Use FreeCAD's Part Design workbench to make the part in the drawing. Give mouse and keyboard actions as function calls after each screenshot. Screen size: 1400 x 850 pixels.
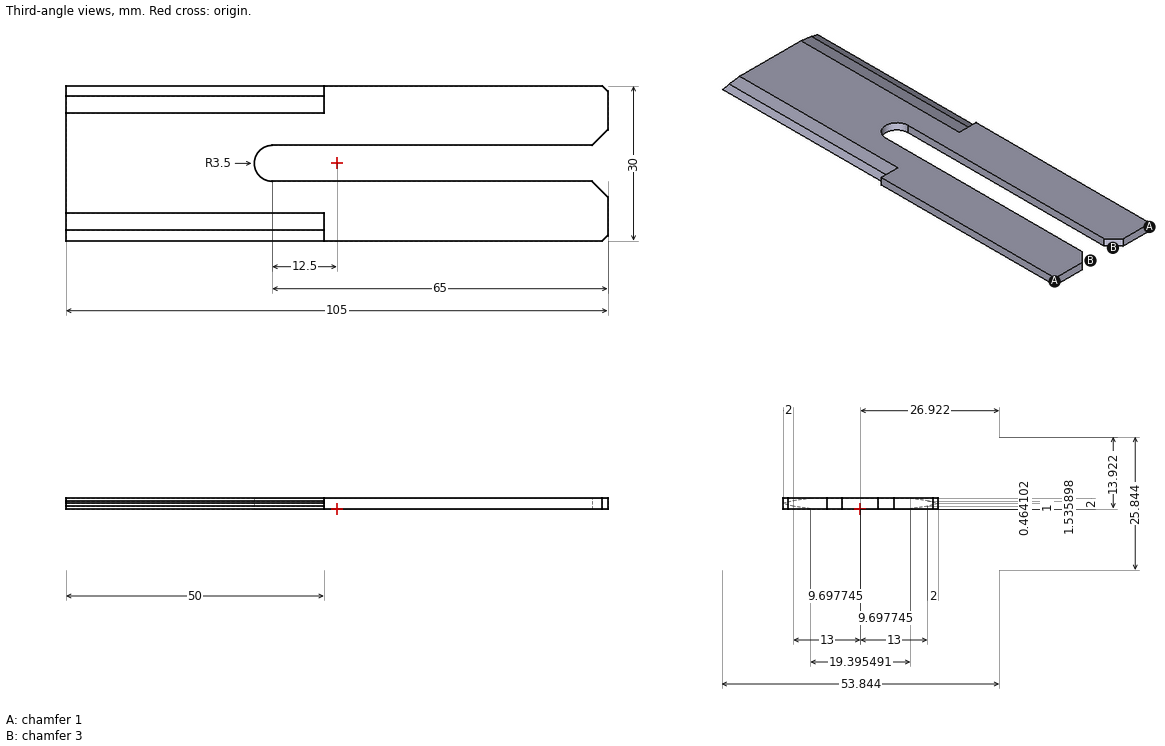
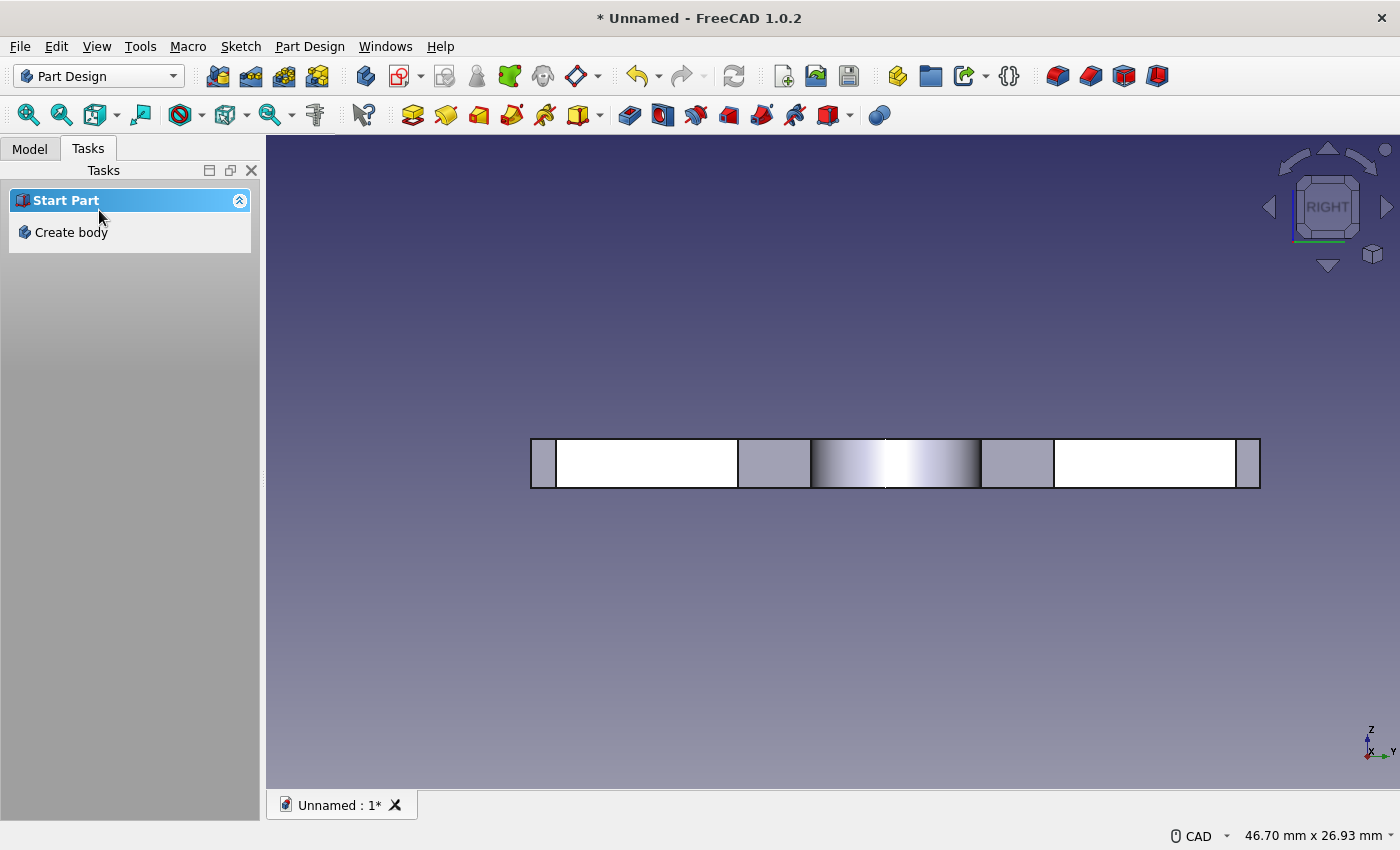
key(0)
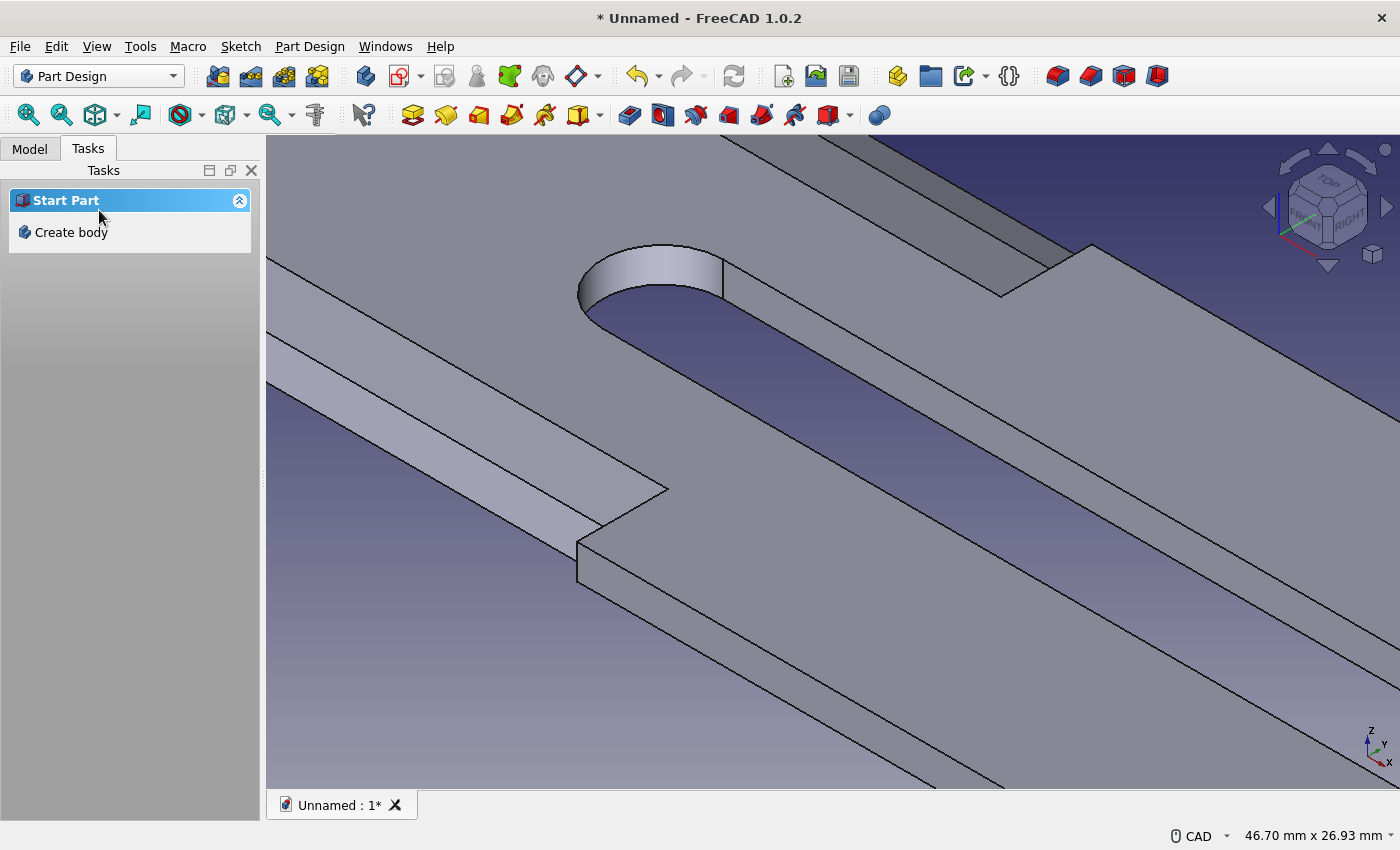
click(29, 116)